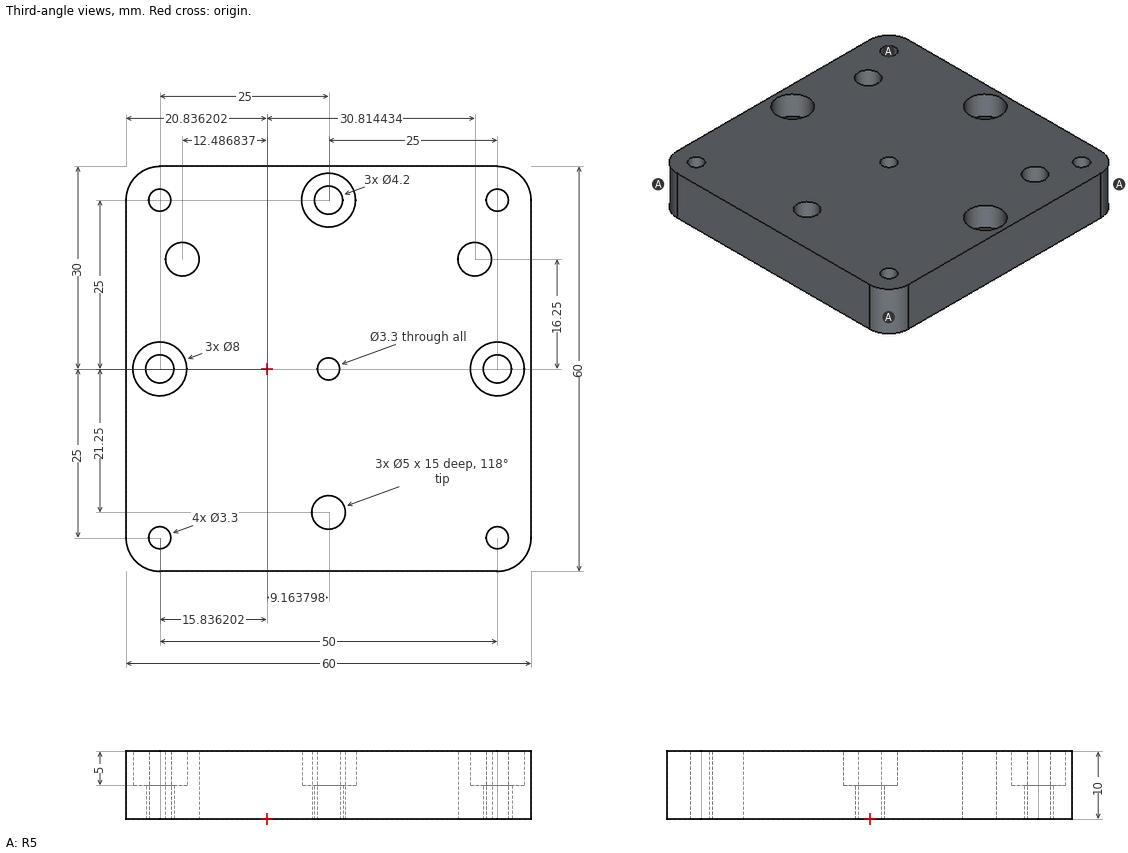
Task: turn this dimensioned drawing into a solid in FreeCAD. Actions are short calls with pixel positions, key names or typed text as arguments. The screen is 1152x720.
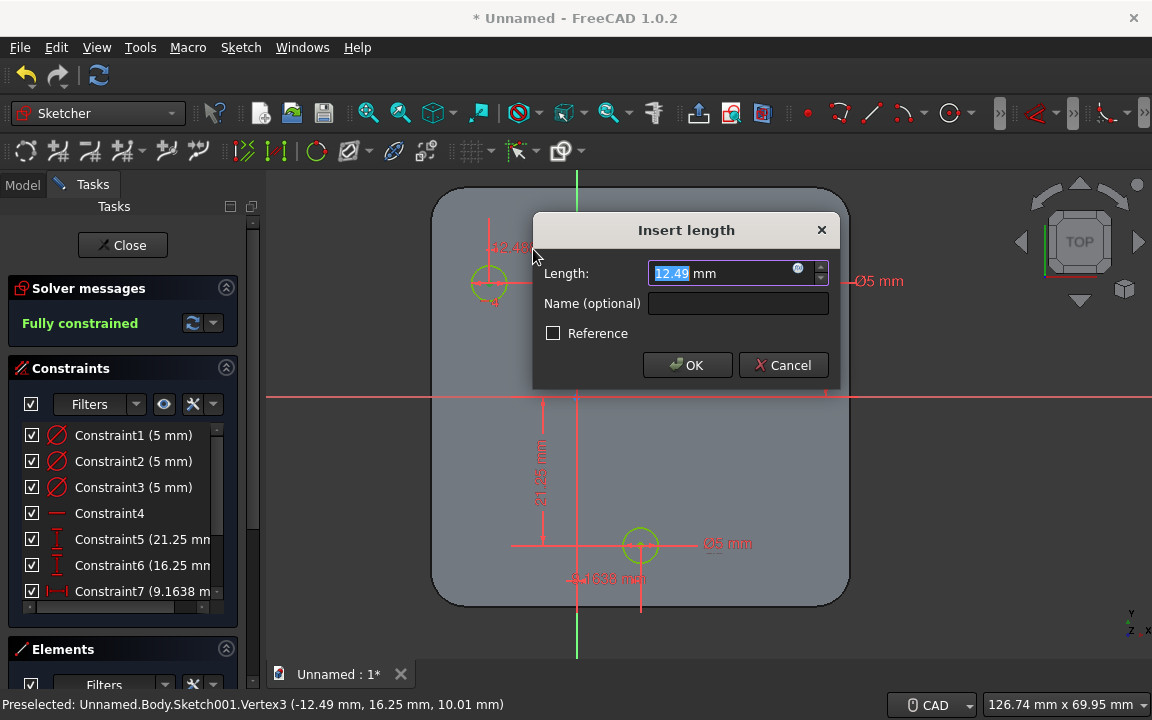
text(12.486837)
key(Return)
key(Escape)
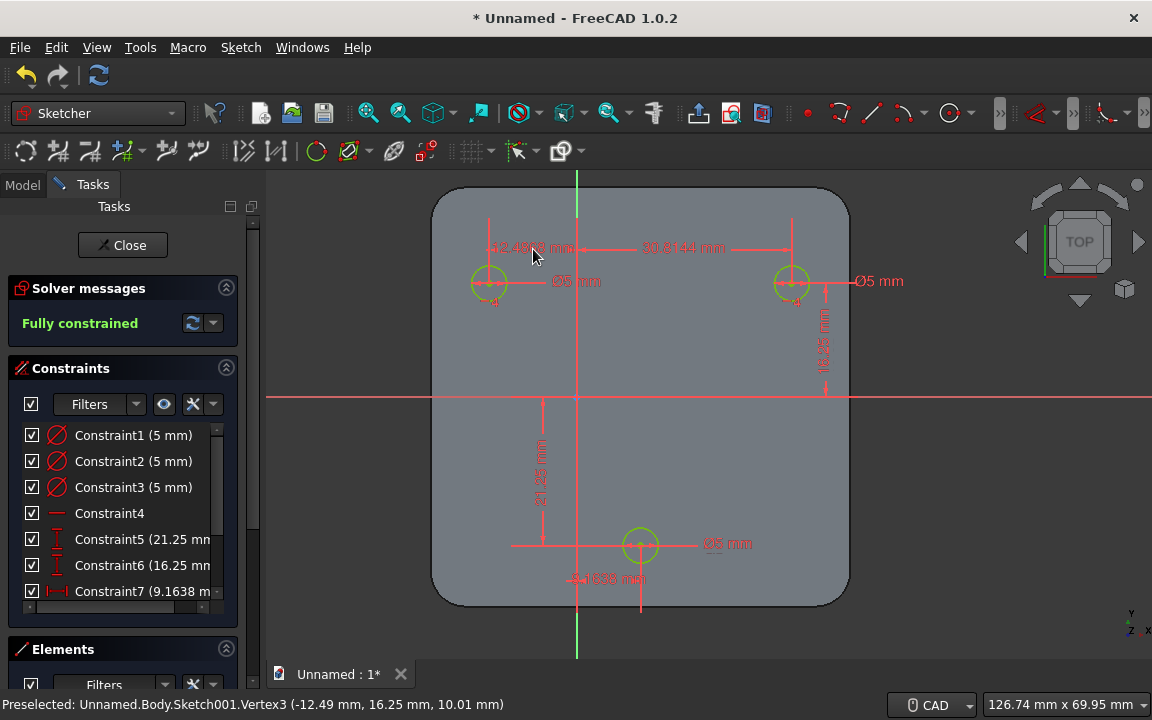
click(123, 245)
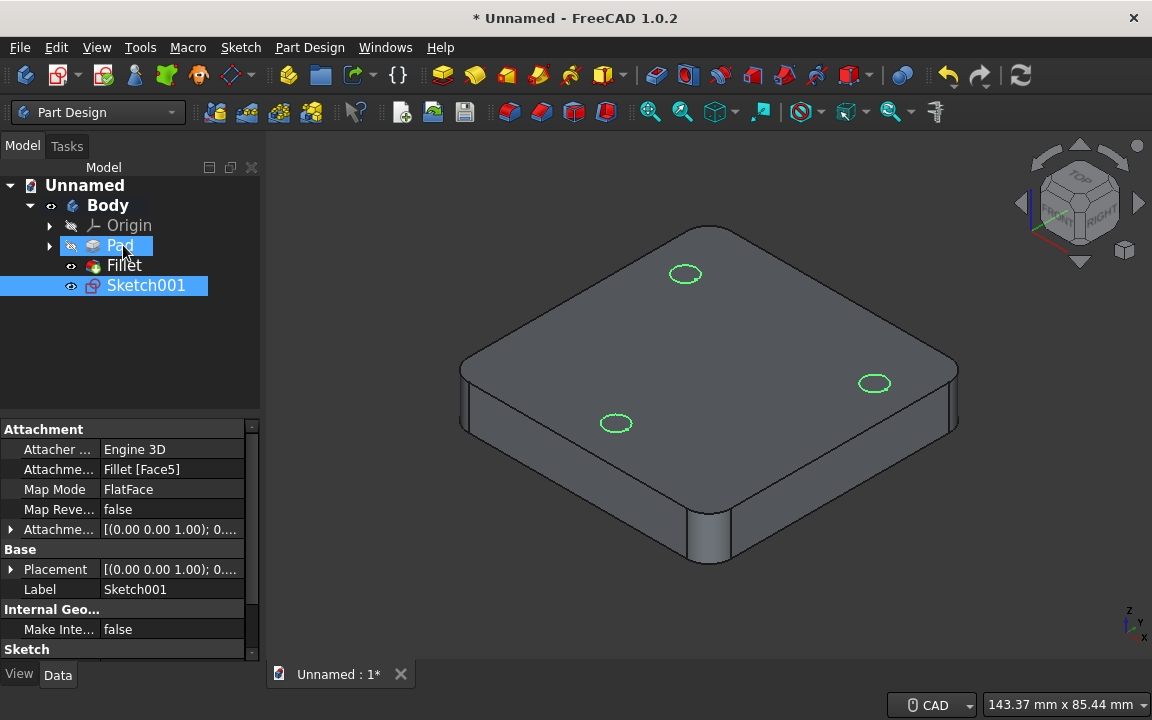
click(690, 76)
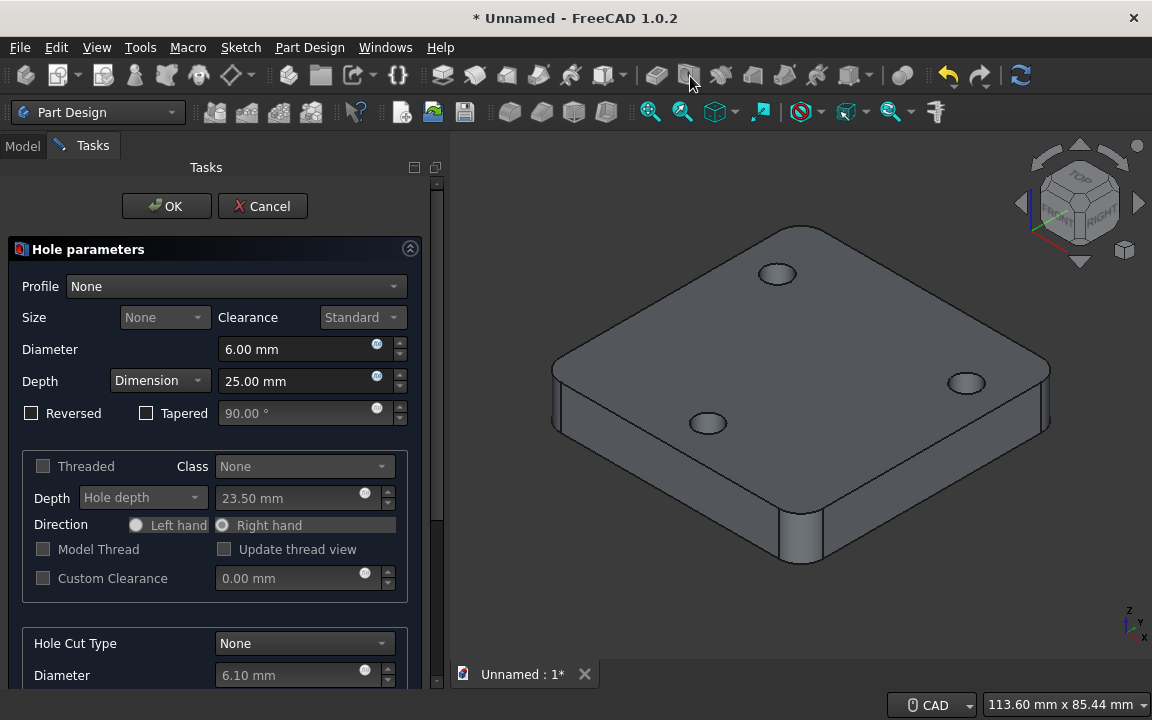
triple_click(305, 349)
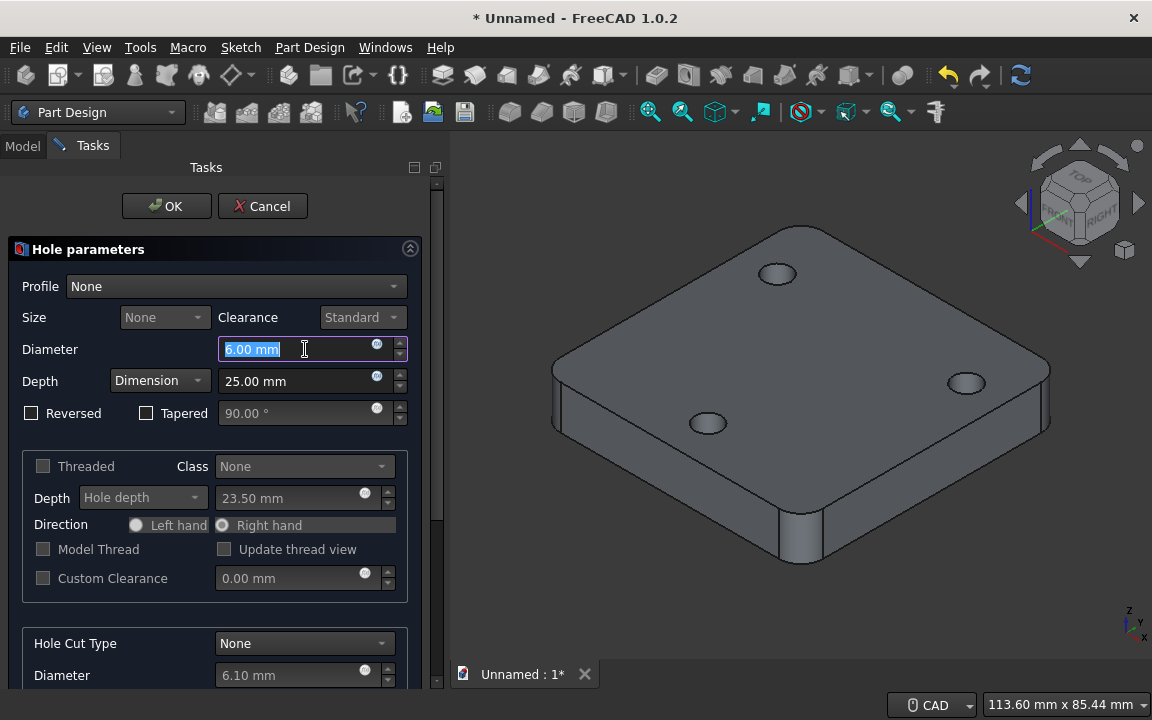
text(5)
key(Tab)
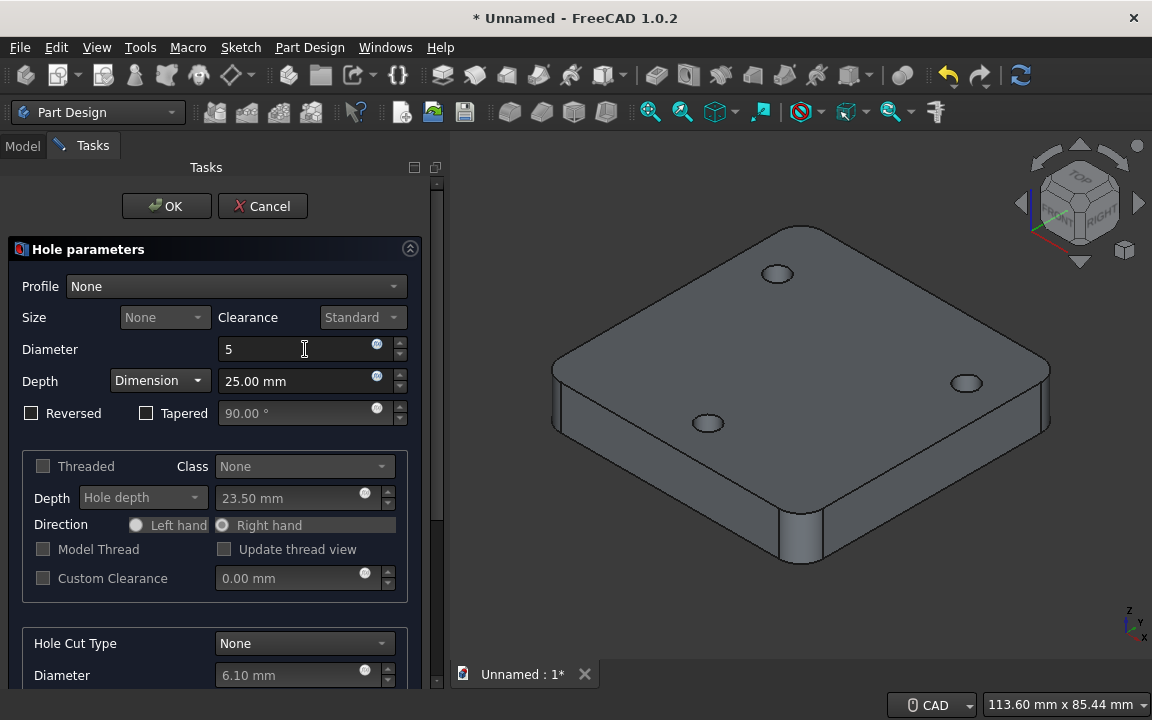
triple_click(305, 381)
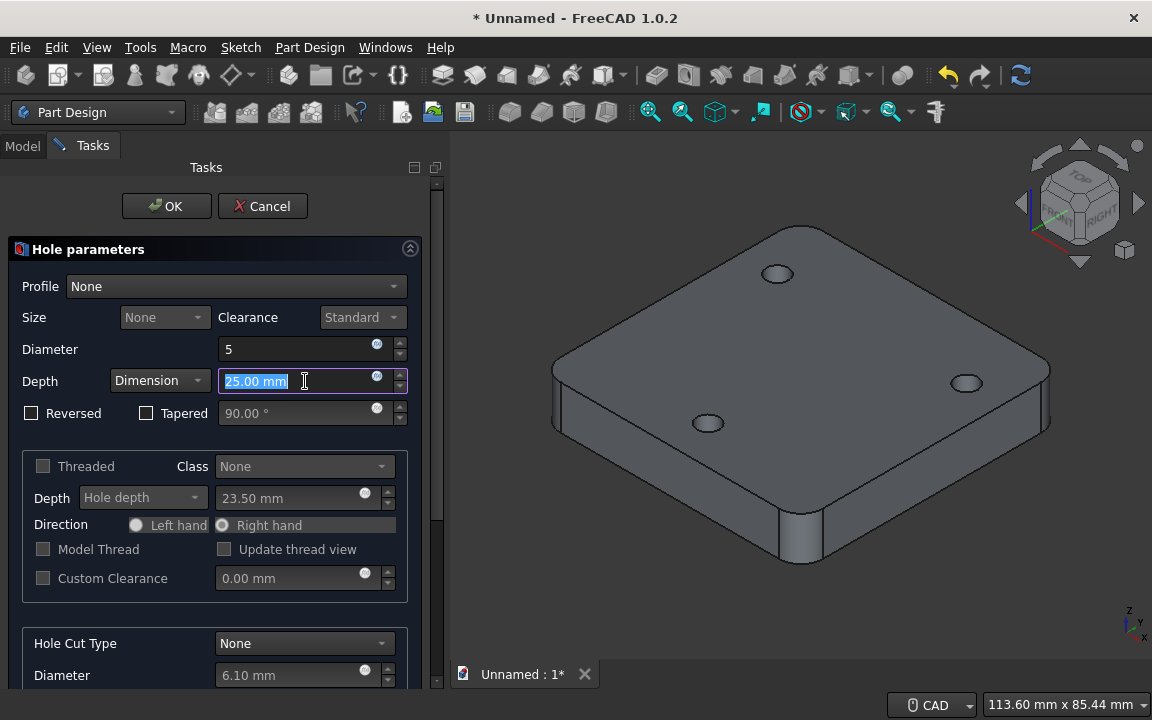
text(15)
key(Tab)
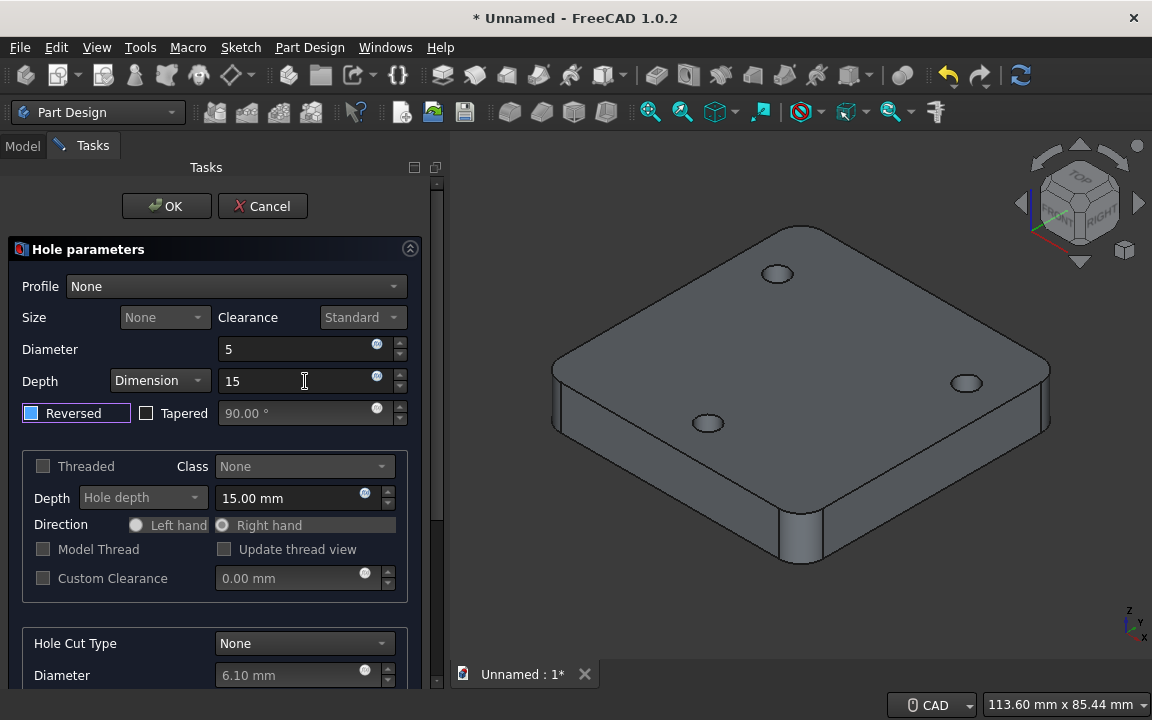
click(167, 206)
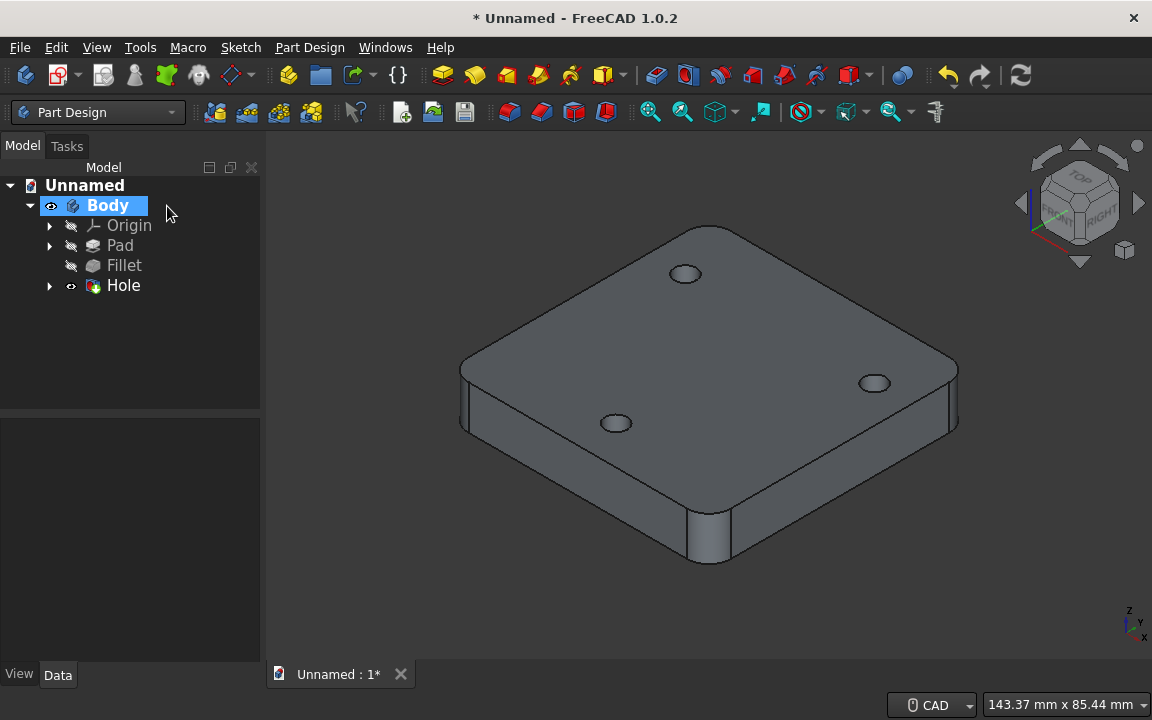
click(746, 347)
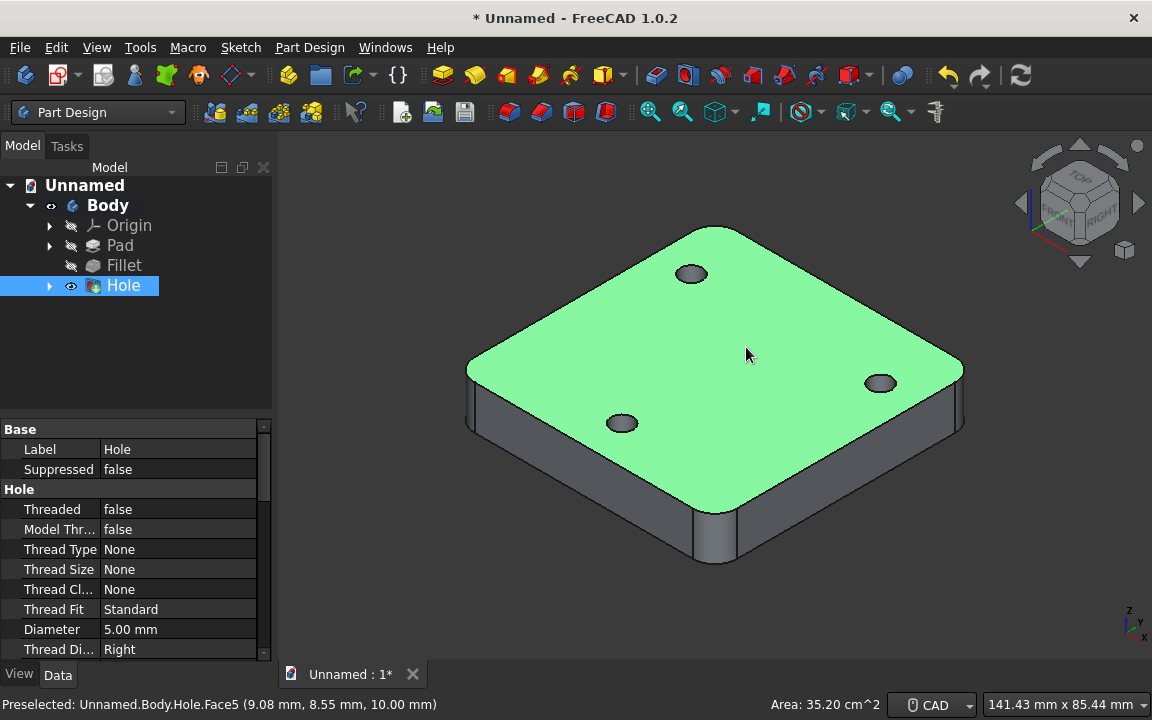
click(58, 76)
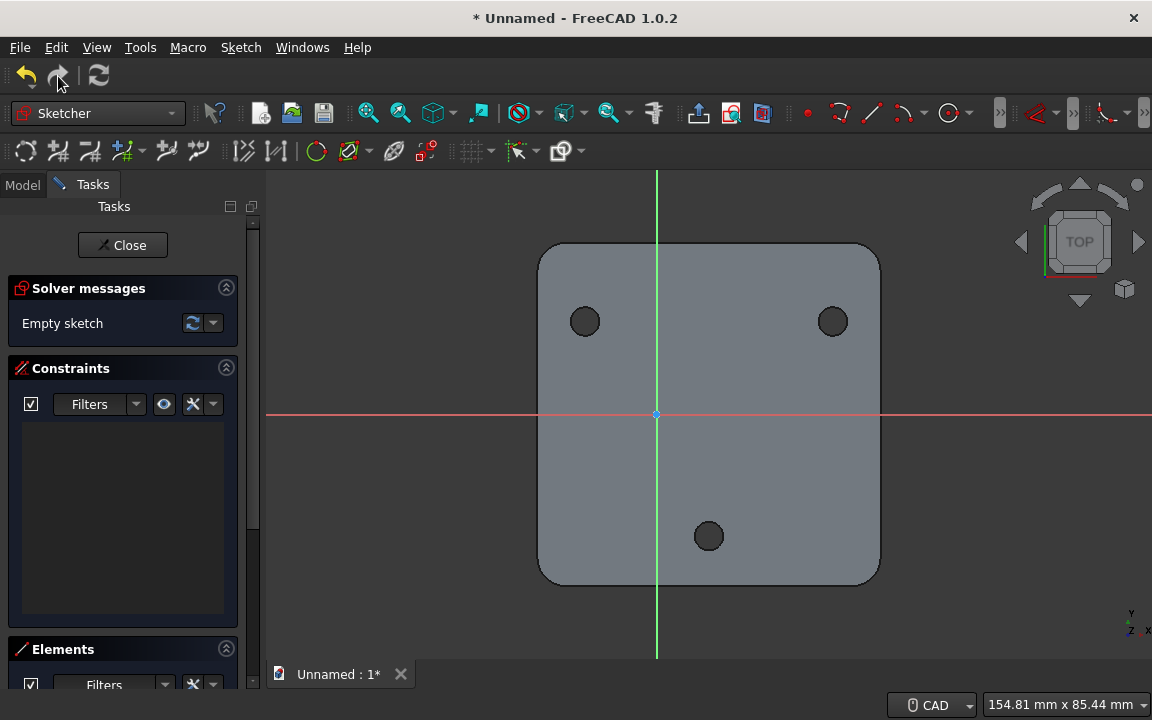
scroll(848, 198, up, 2)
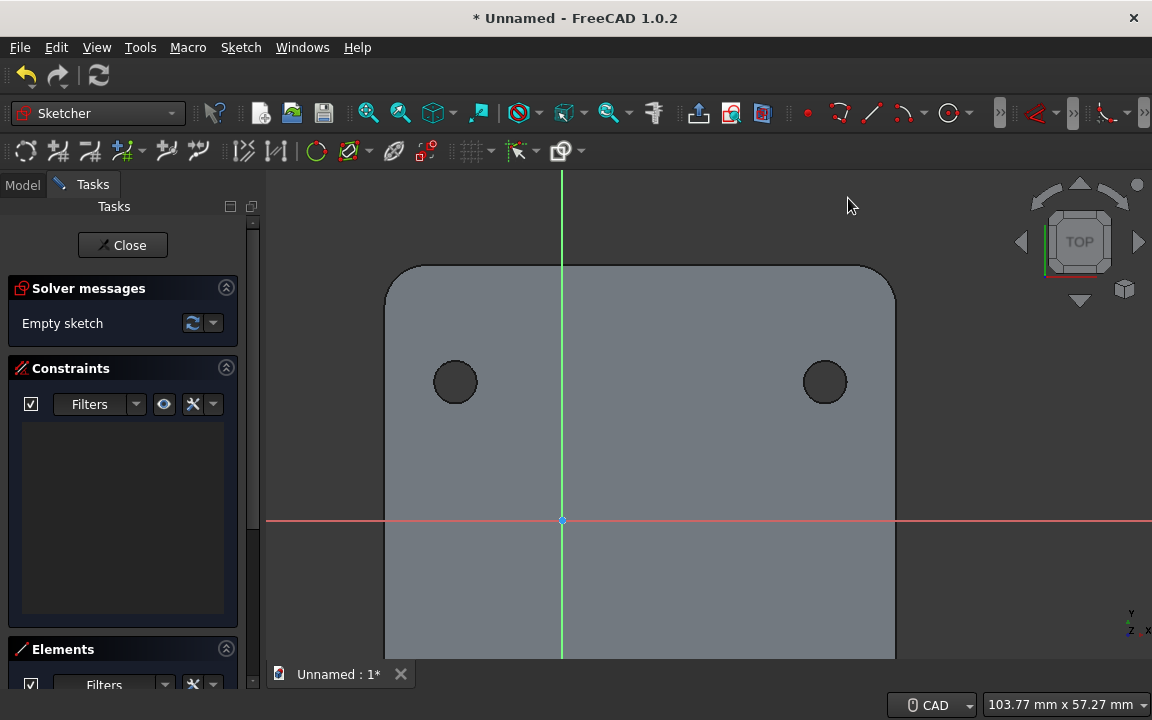
key(g)
key(c)